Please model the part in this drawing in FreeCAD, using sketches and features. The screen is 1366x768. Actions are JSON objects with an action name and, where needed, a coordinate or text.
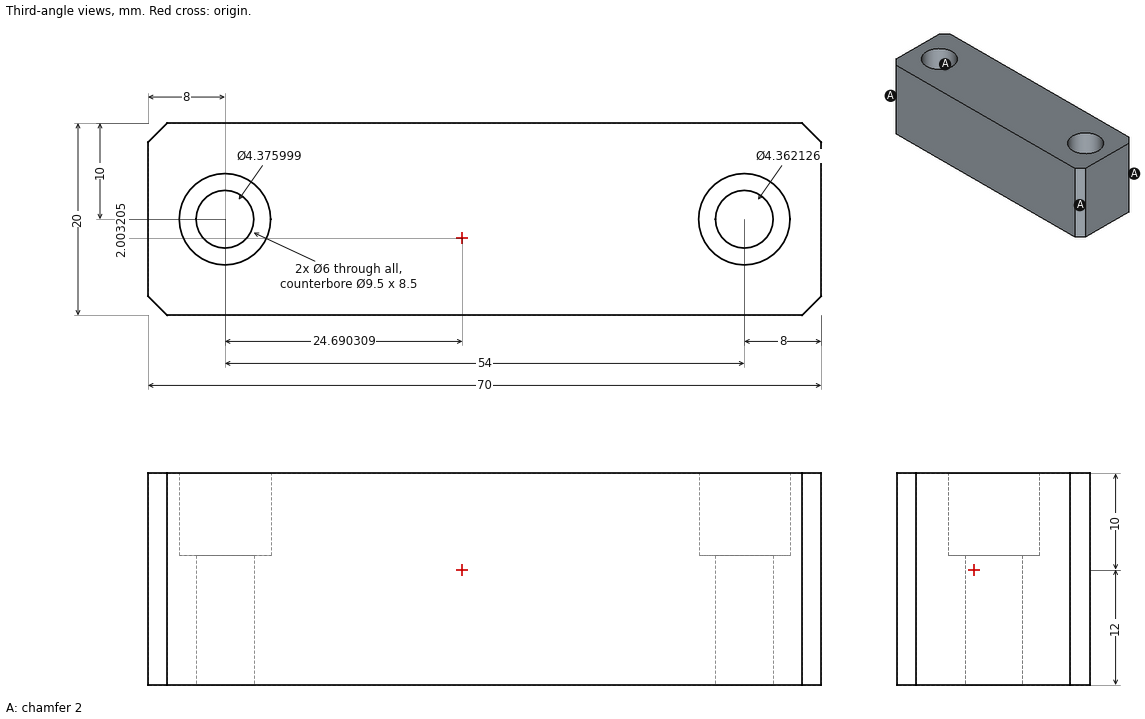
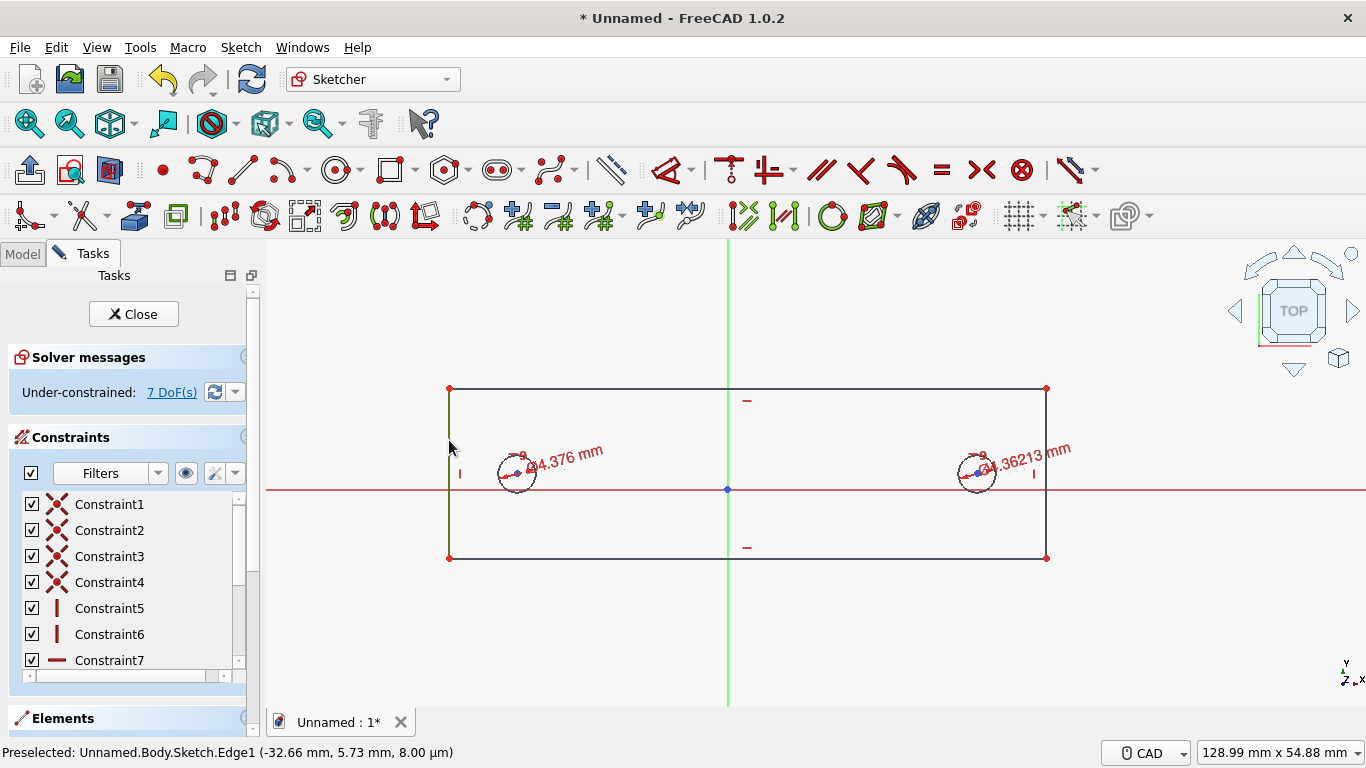
{"action": "key", "text": "i"}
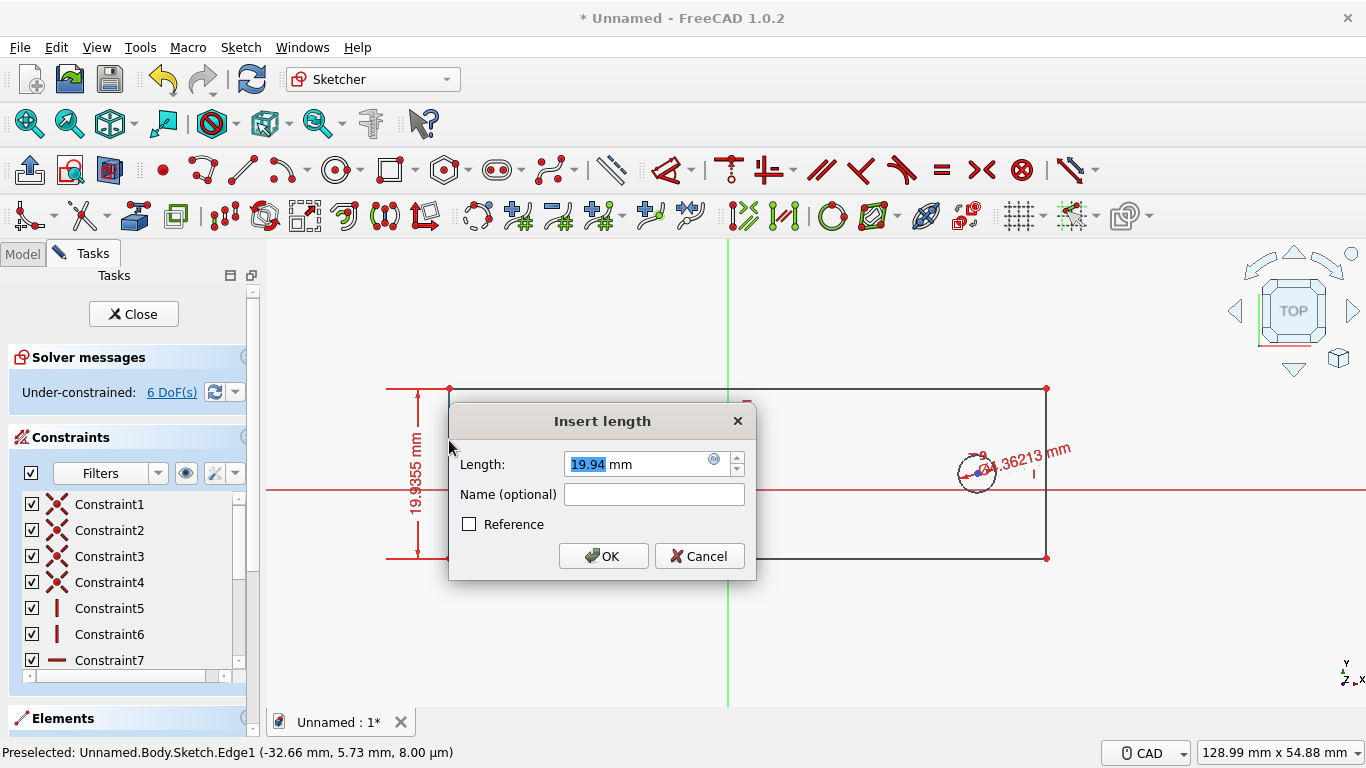
{"action": "type", "text": "20"}
{"action": "key", "text": "Return"}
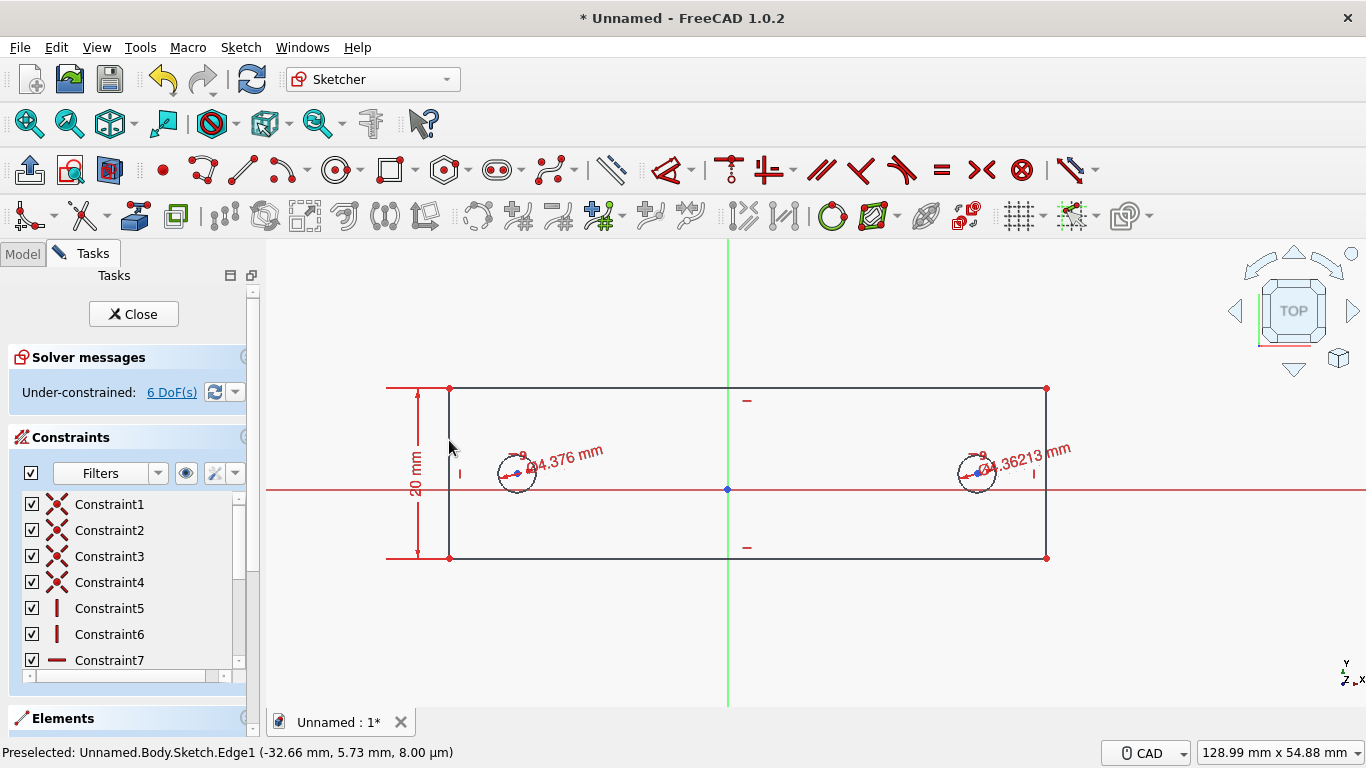
{"action": "left_click", "coordinate": [628, 559]}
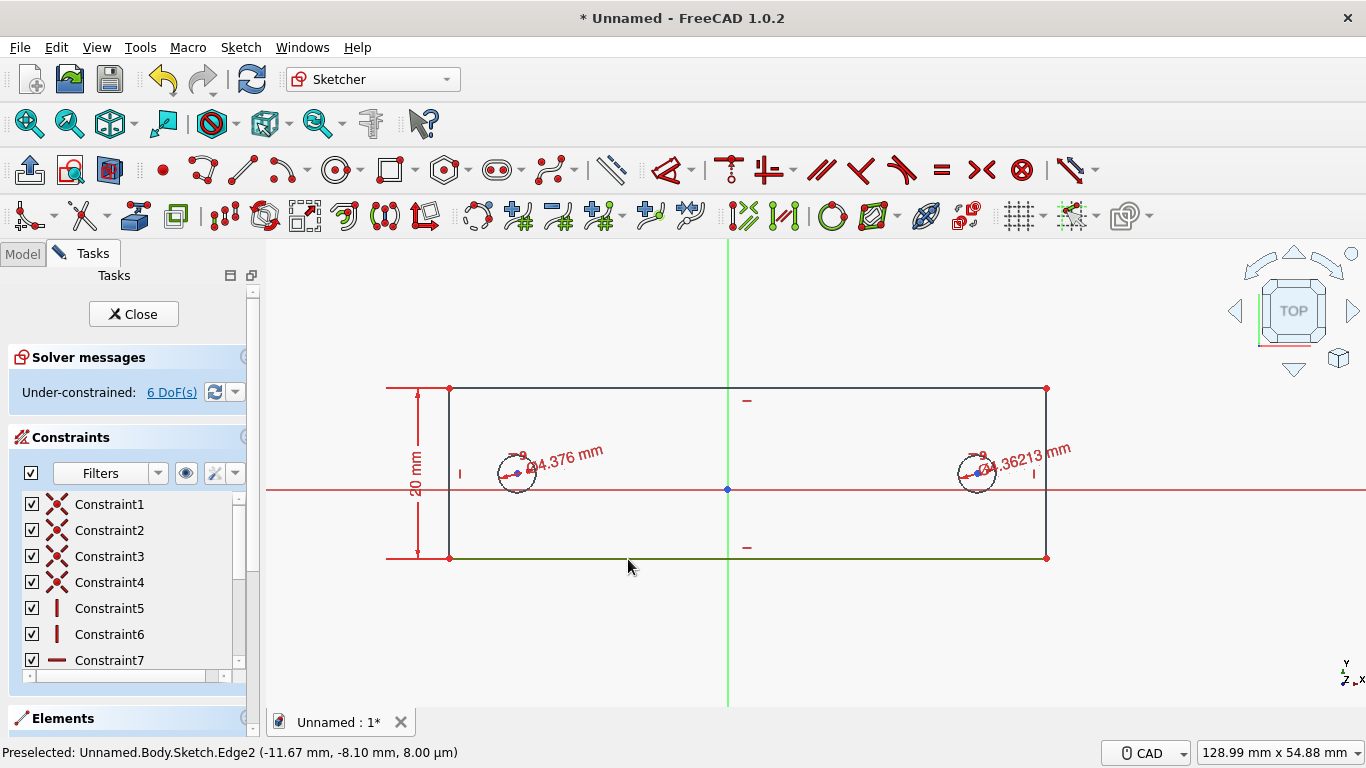
{"action": "key", "text": "l"}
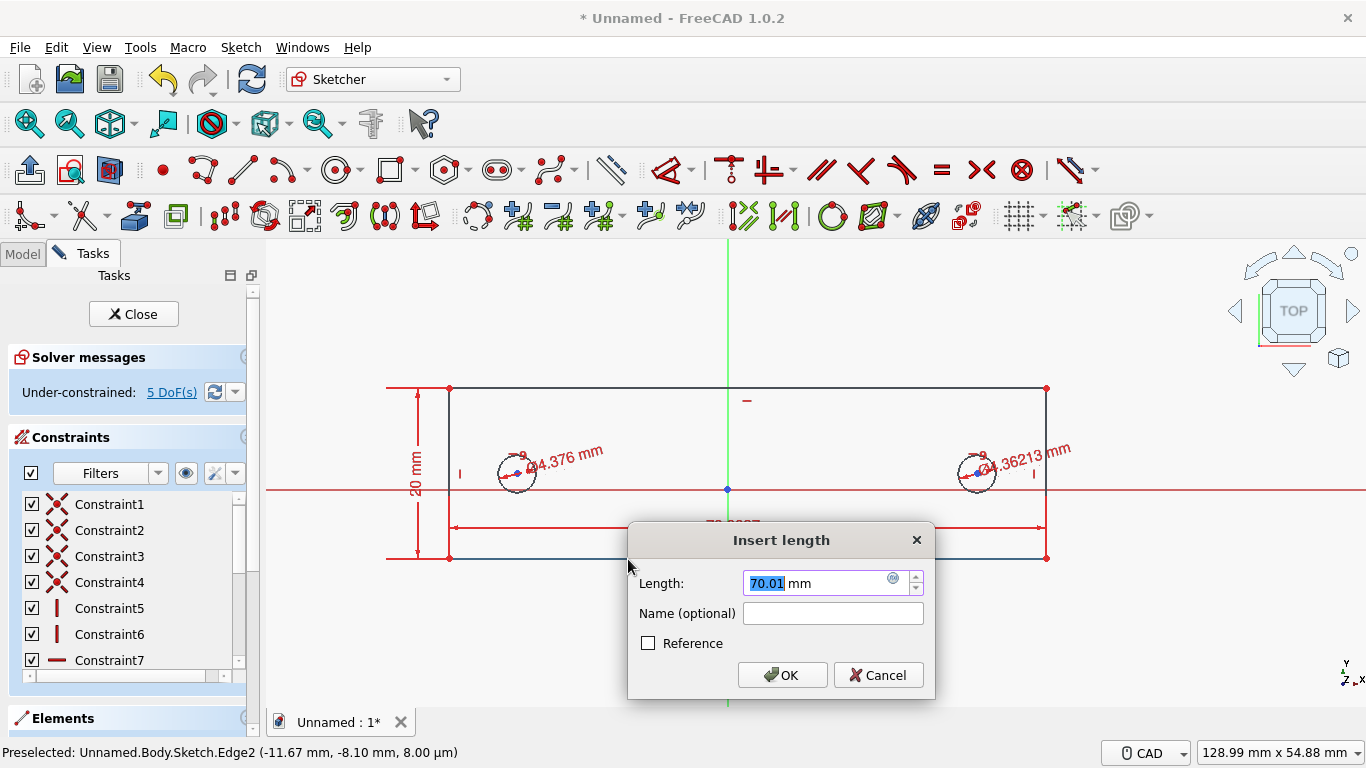
{"action": "type", "text": "70"}
{"action": "key", "text": "Return"}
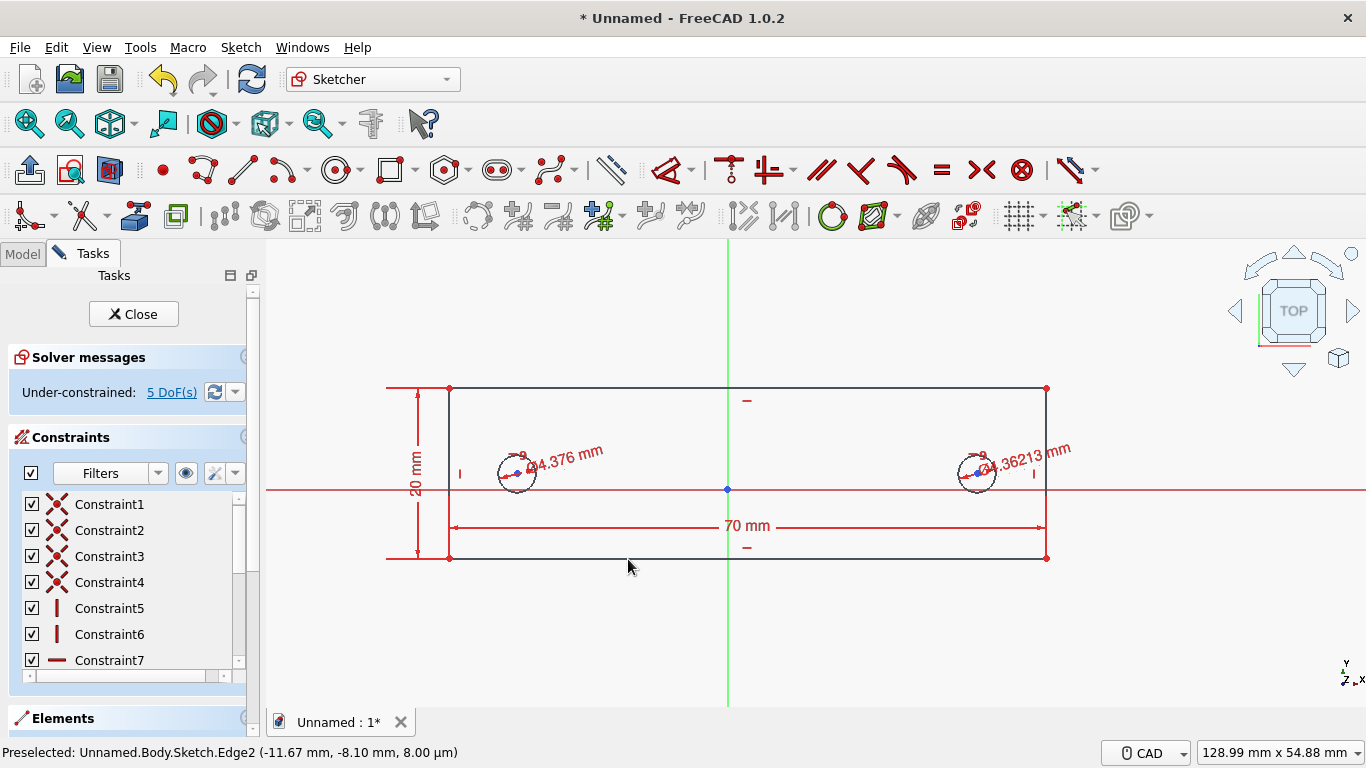
{"action": "left_click", "coordinate": [449, 388]}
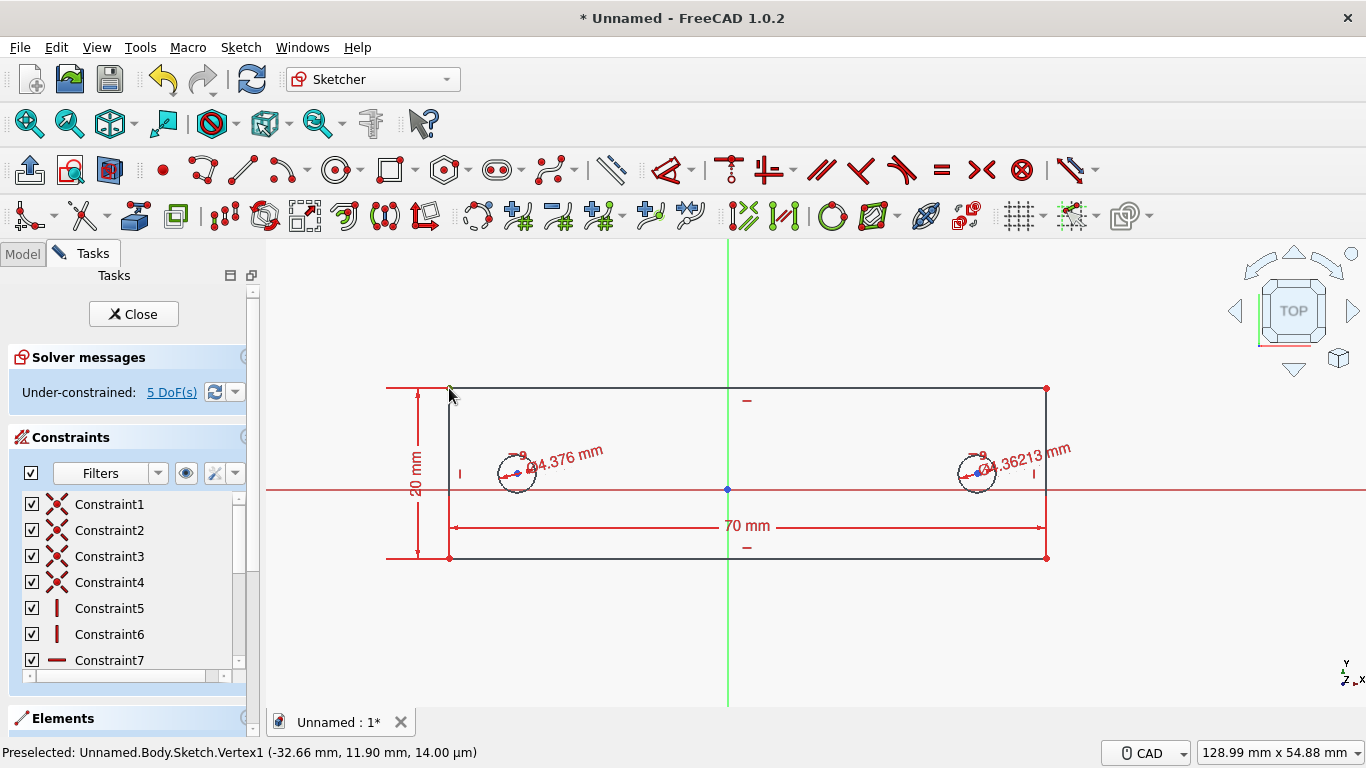
{"action": "left_click", "coordinate": [517, 474]}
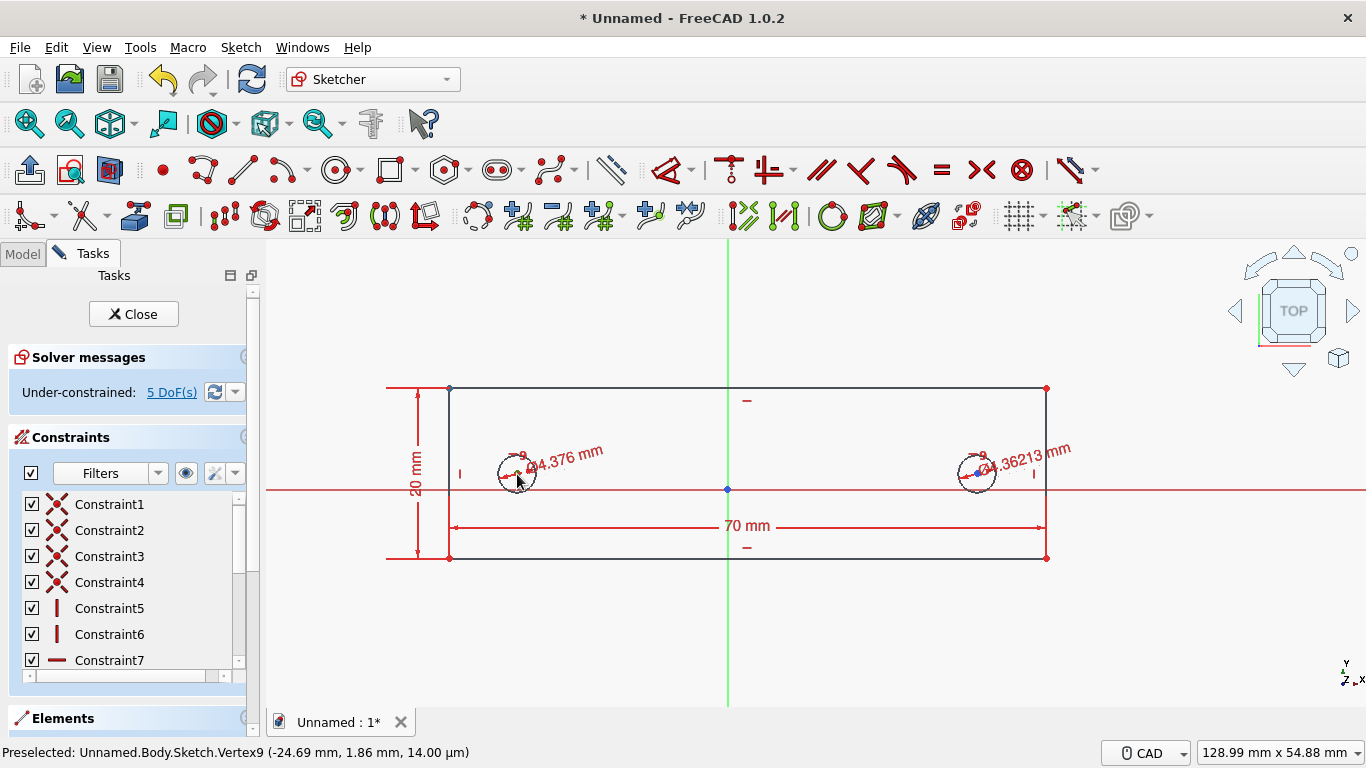
{"action": "key", "text": "l"}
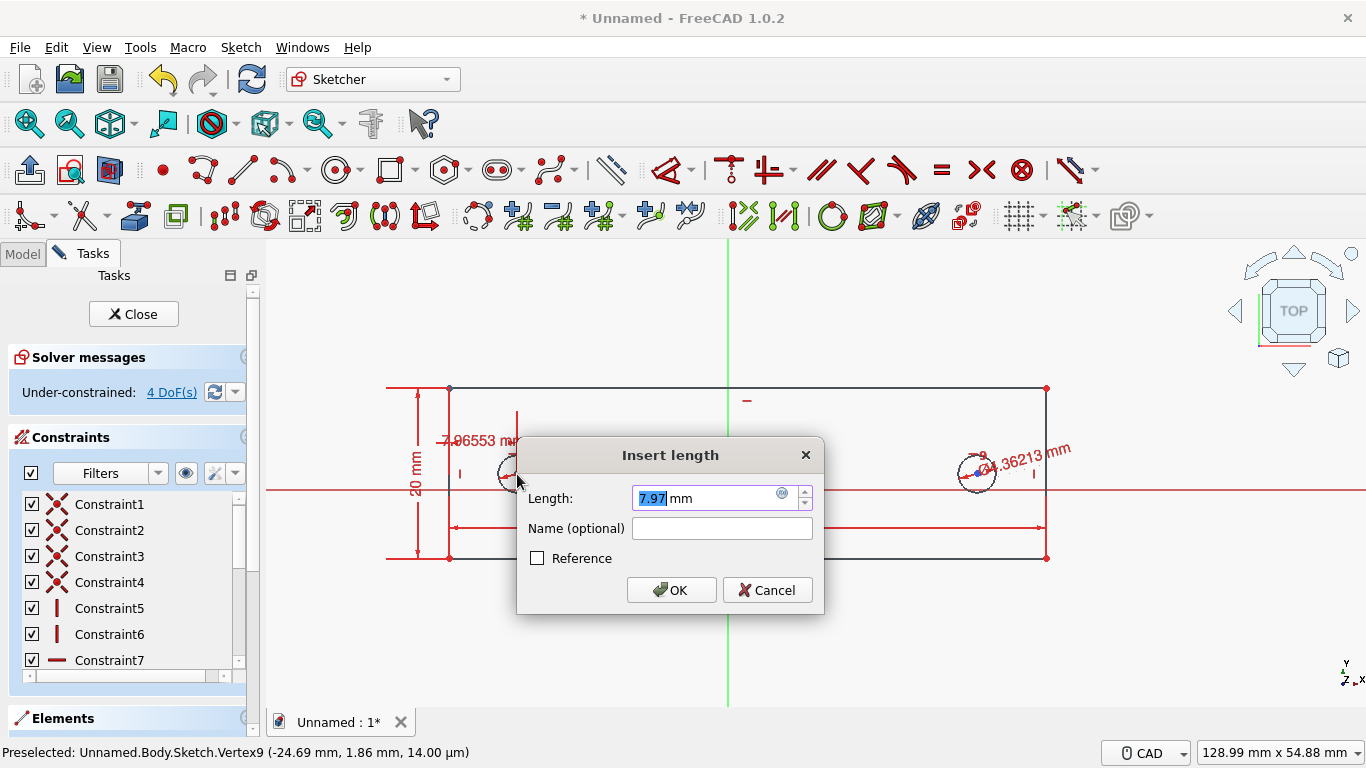
{"action": "type", "text": "8"}
{"action": "key", "text": "Return"}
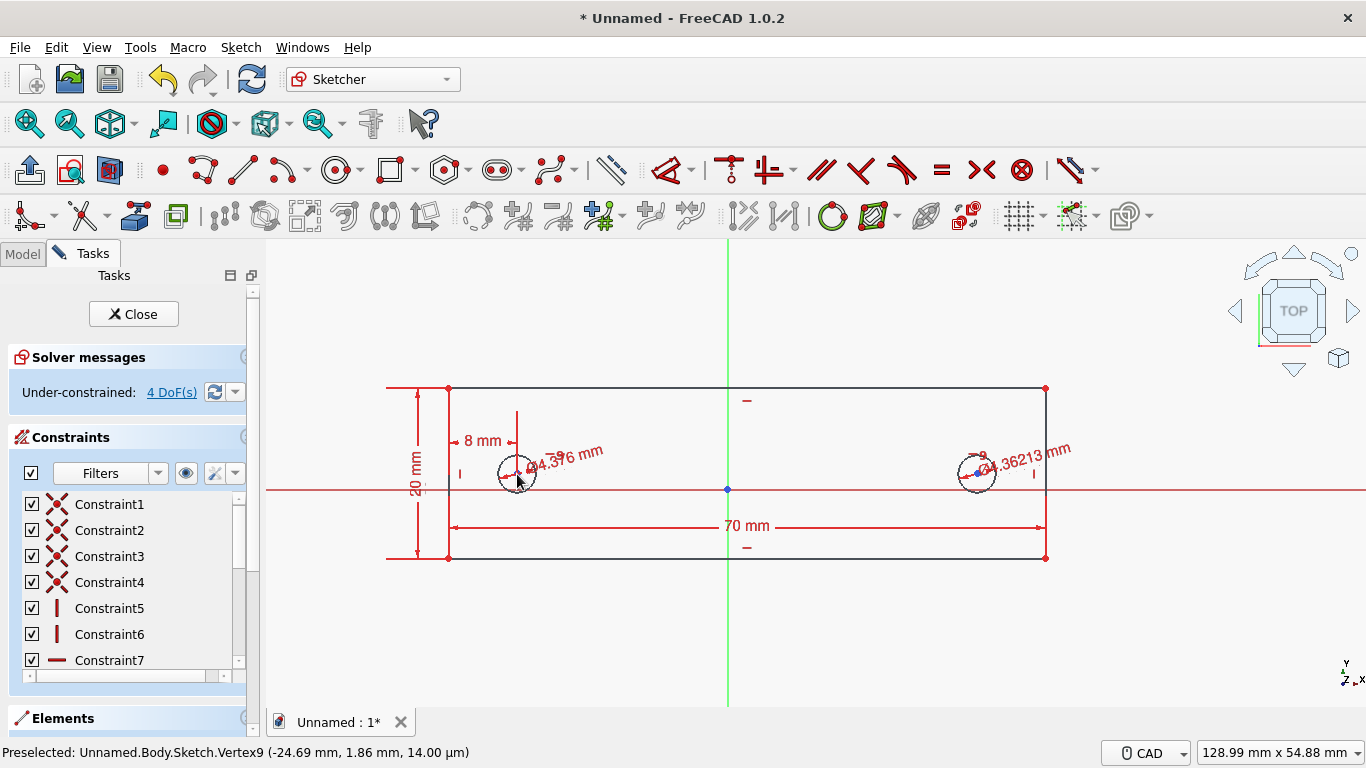
{"action": "left_click", "coordinate": [1046, 559]}